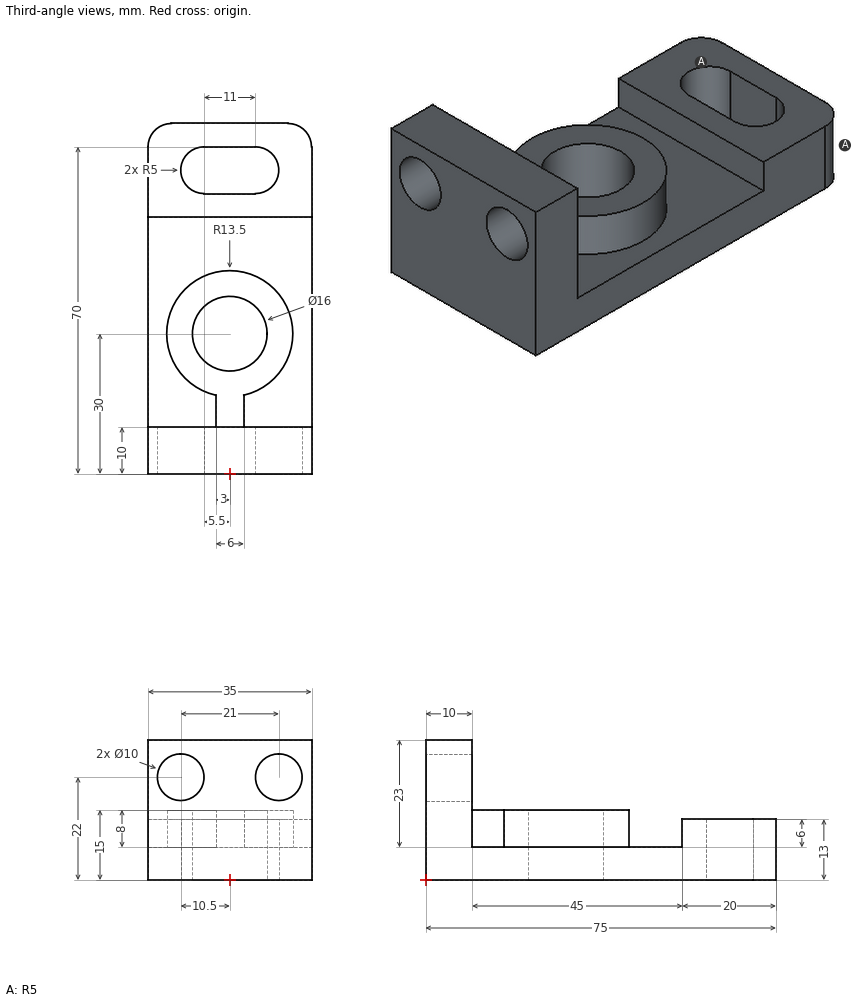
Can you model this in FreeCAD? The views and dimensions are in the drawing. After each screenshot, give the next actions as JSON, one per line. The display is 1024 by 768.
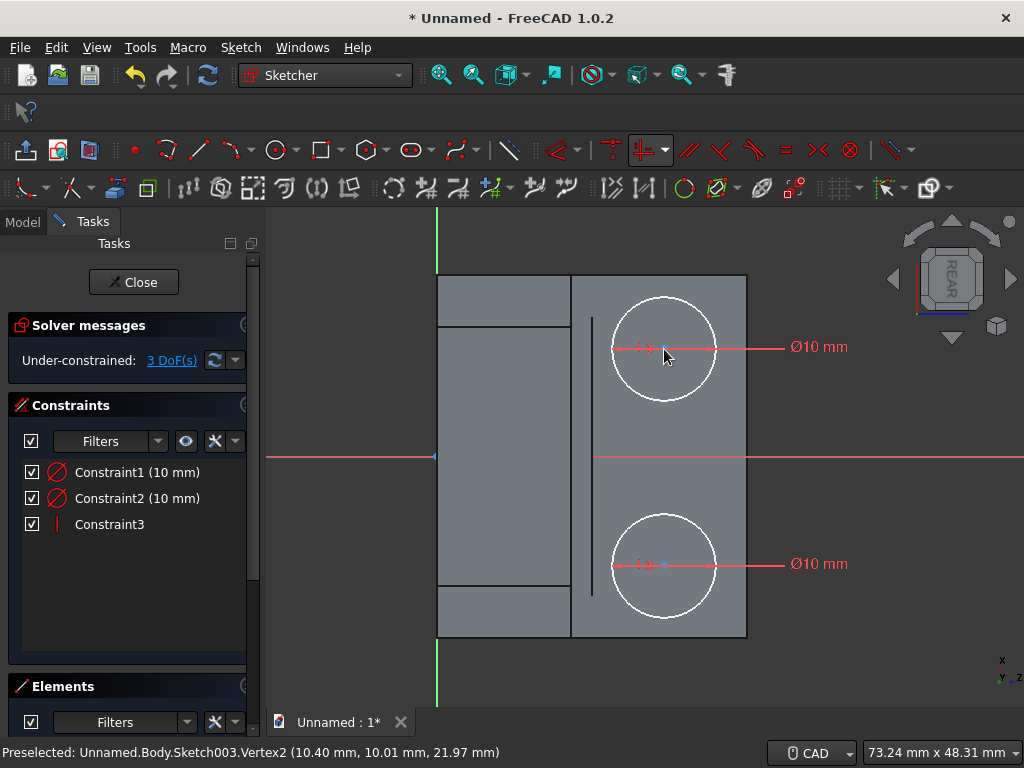
{"action": "key", "text": "d"}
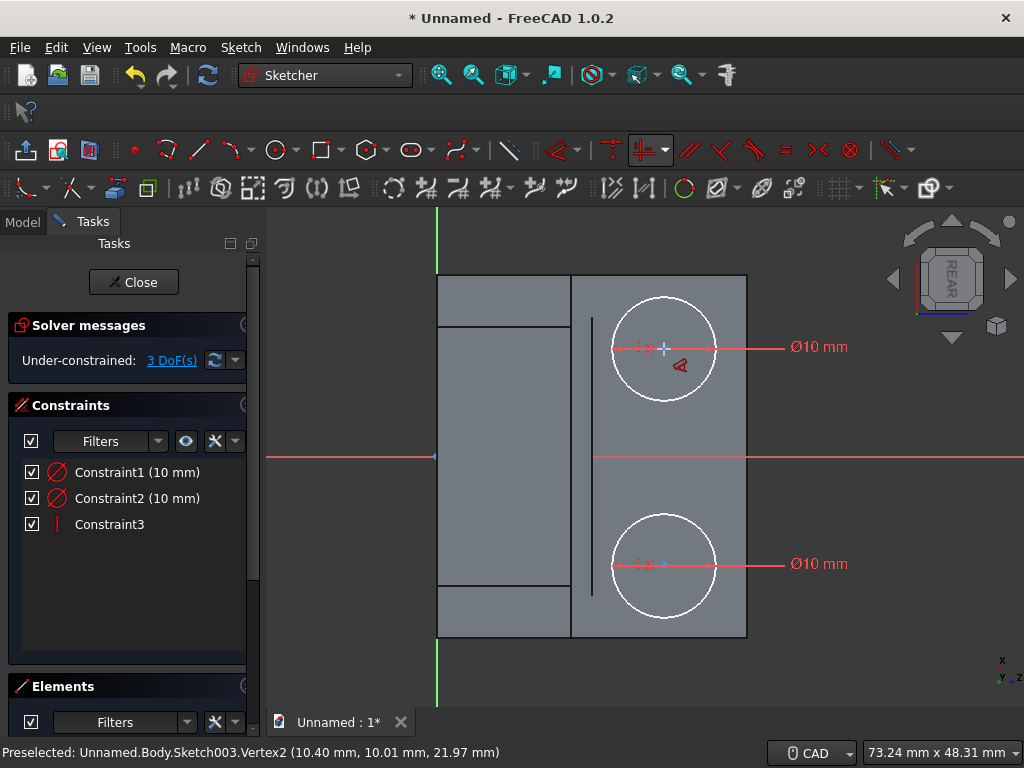
{"action": "left_click", "coordinate": [664, 566]}
{"action": "left_click", "coordinate": [550, 600]}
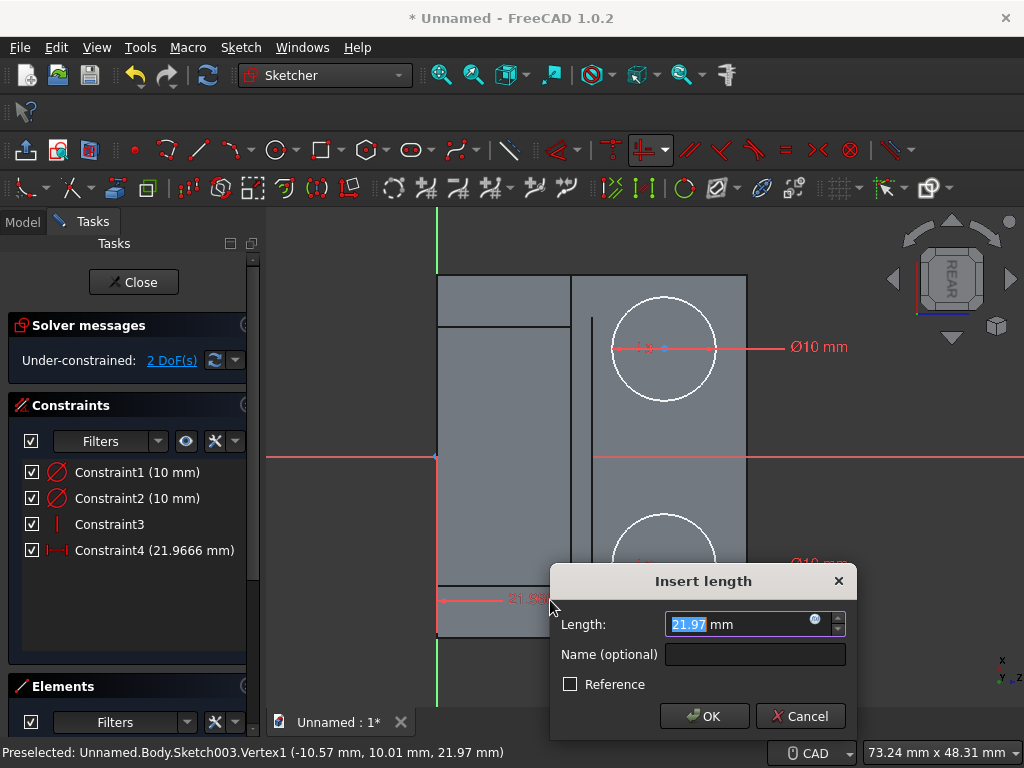
{"action": "type", "text": "22"}
{"action": "key", "text": "Return"}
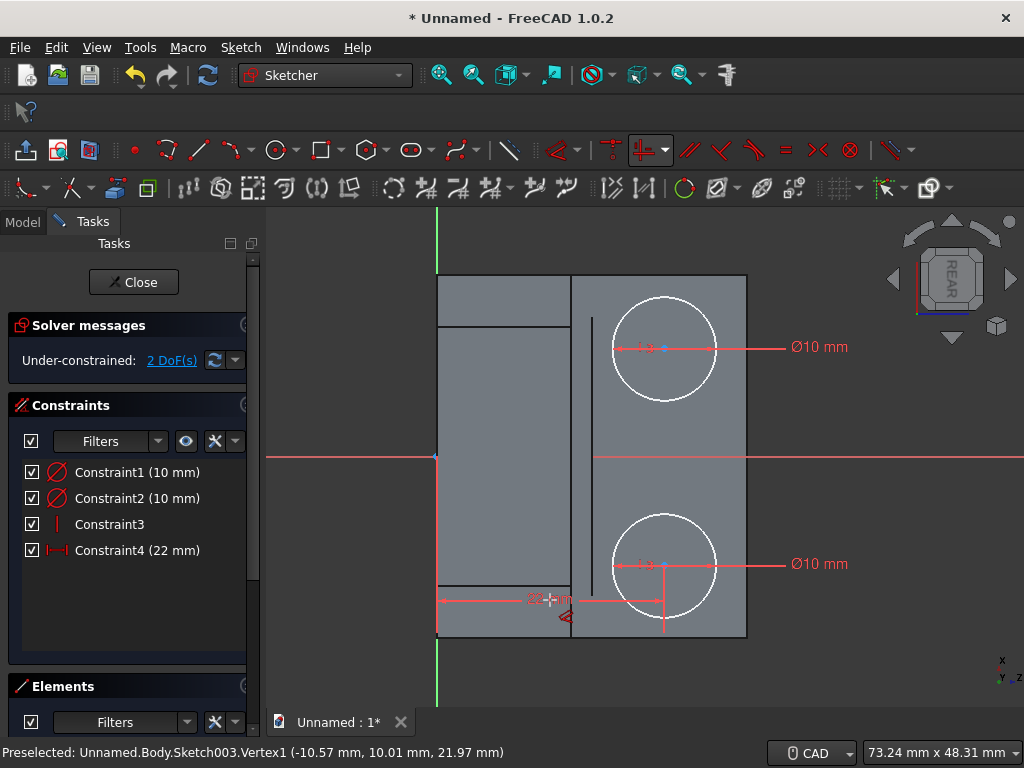
{"action": "left_click", "coordinate": [664, 566]}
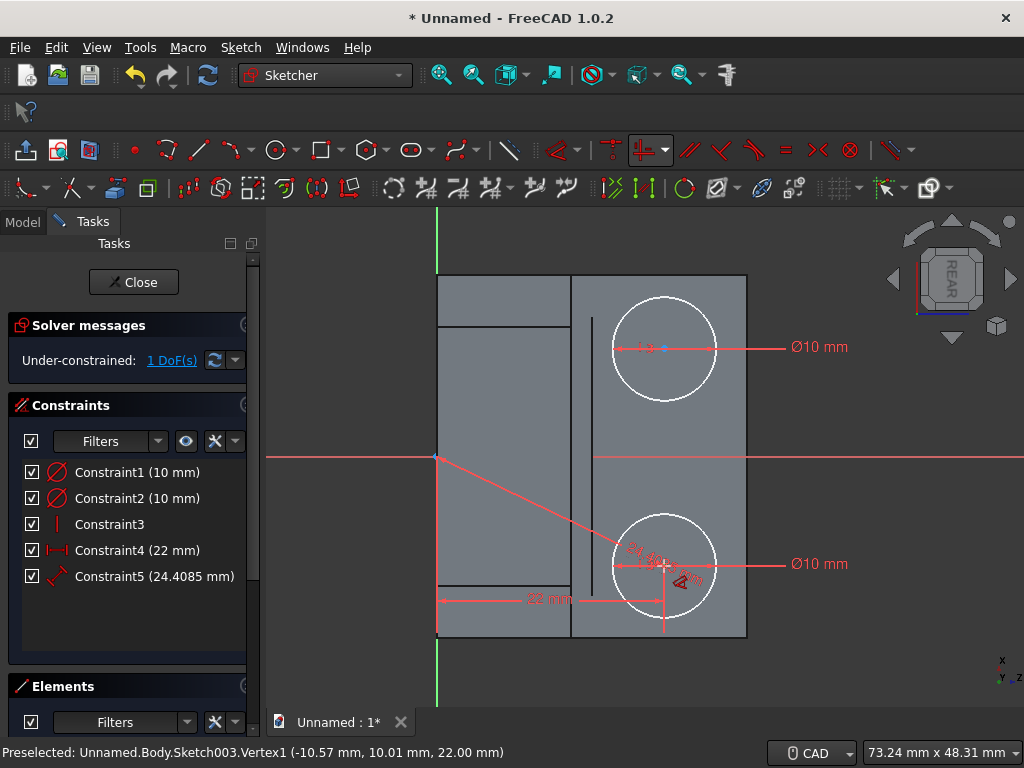
{"action": "left_click", "coordinate": [664, 349]}
{"action": "left_click", "coordinate": [698, 408]}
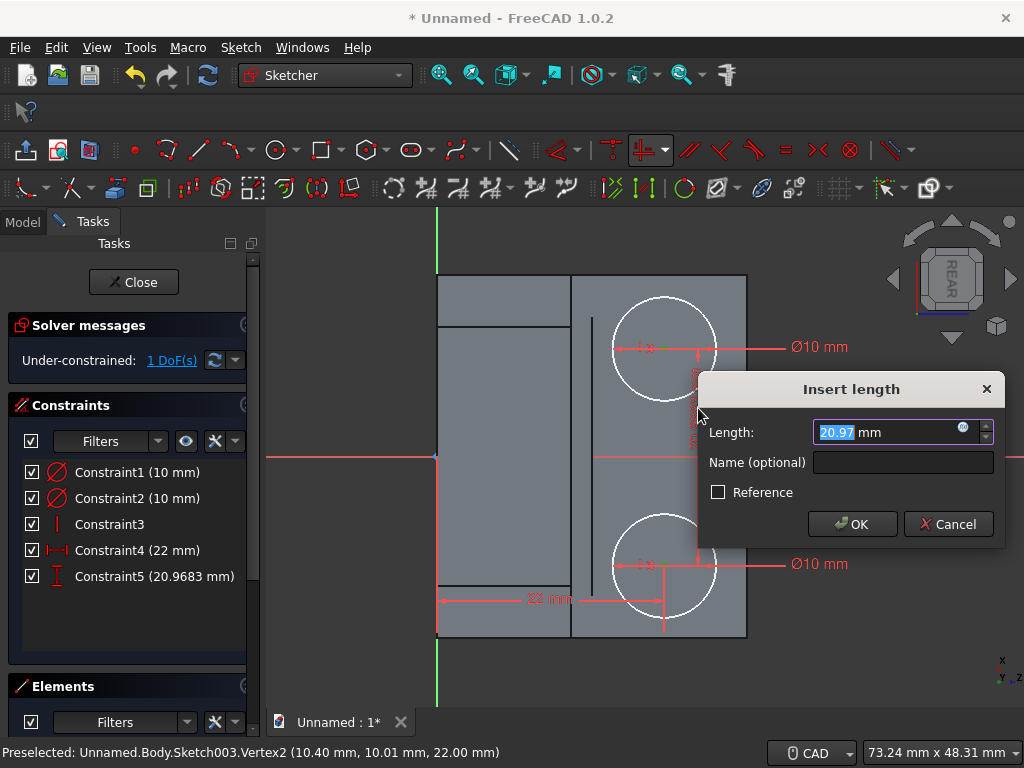
{"action": "type", "text": "21"}
{"action": "key", "text": "Return"}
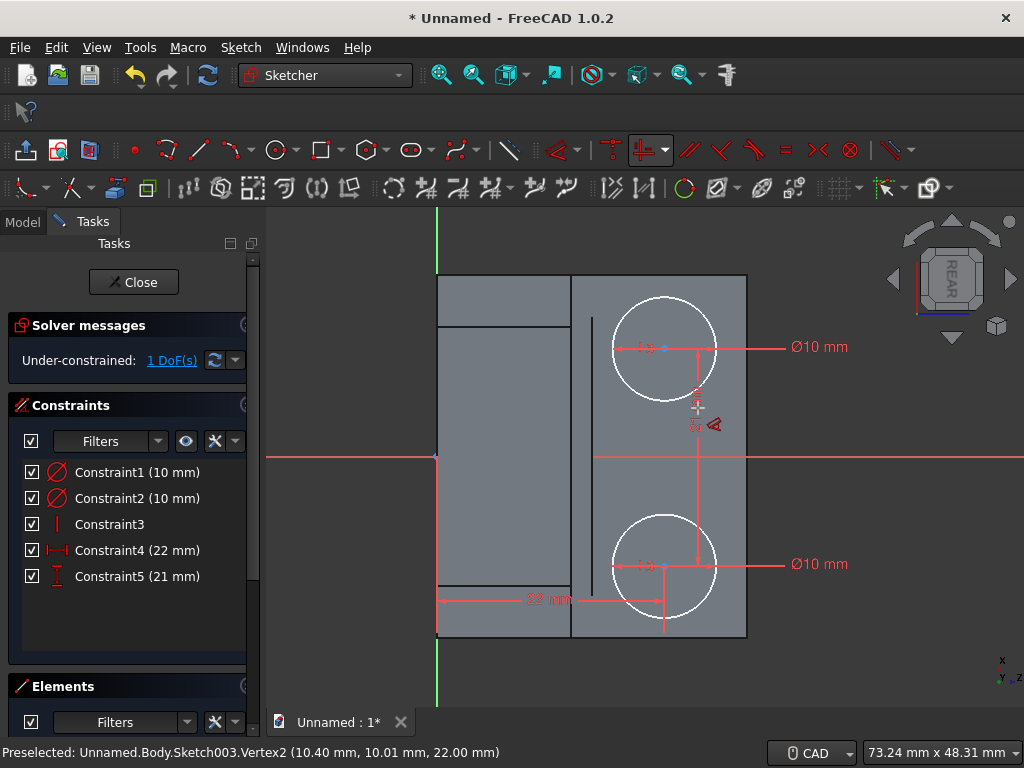
{"action": "left_click", "coordinate": [664, 566]}
{"action": "left_click", "coordinate": [403, 511]}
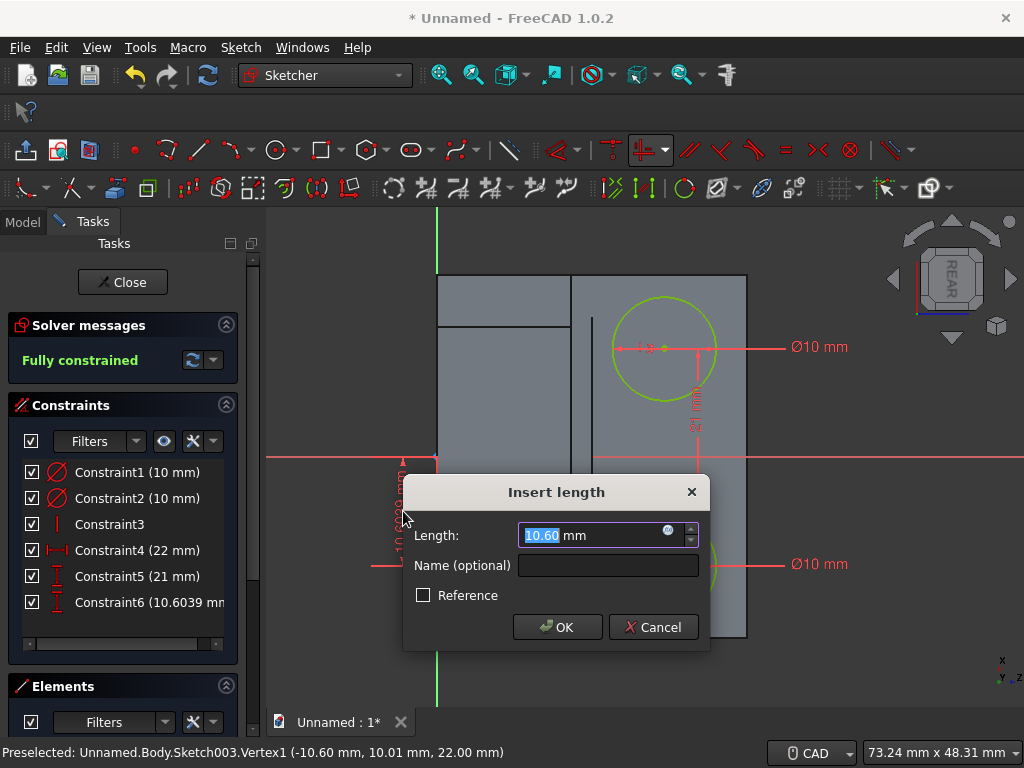
{"action": "type", "text": "10.5"}
{"action": "key", "text": "Return"}
{"action": "key", "text": "Escape"}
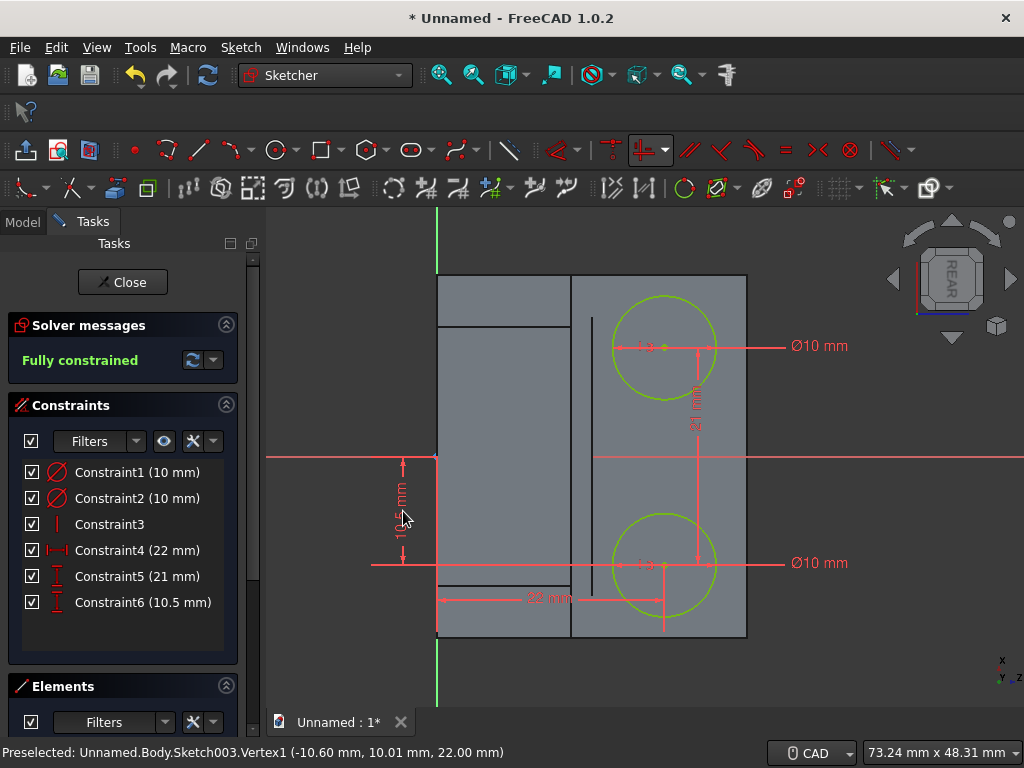
{"action": "left_click", "coordinate": [123, 282]}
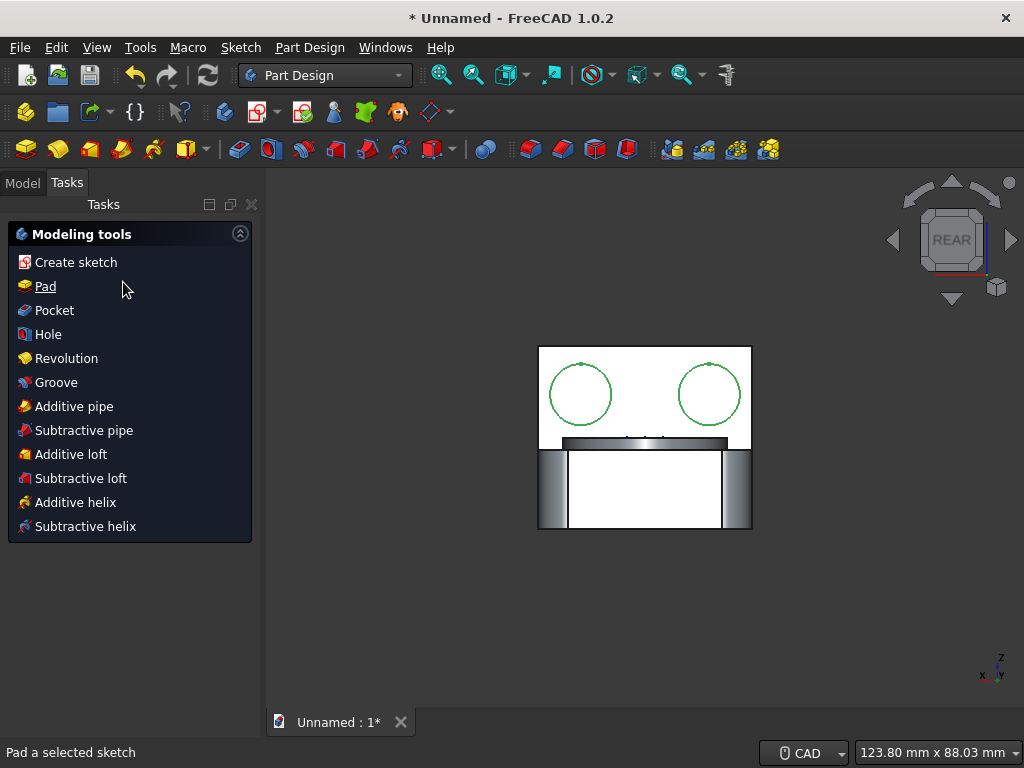
{"action": "left_click", "coordinate": [240, 150]}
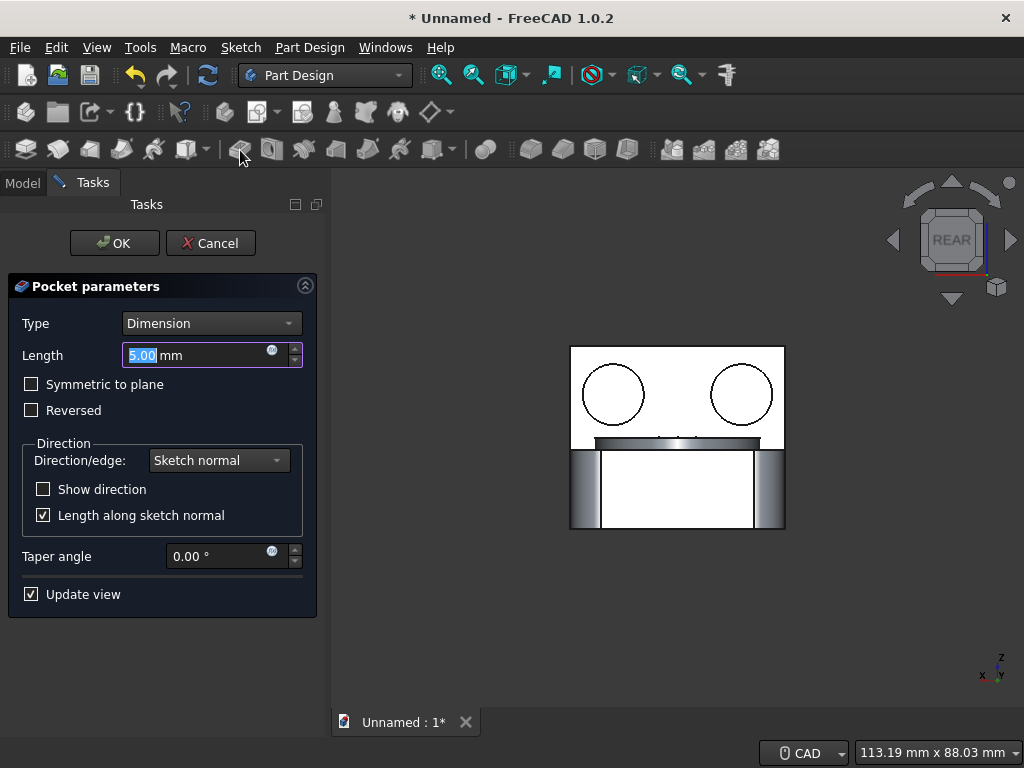
{"action": "type", "text": "10"}
{"action": "key", "text": "Tab"}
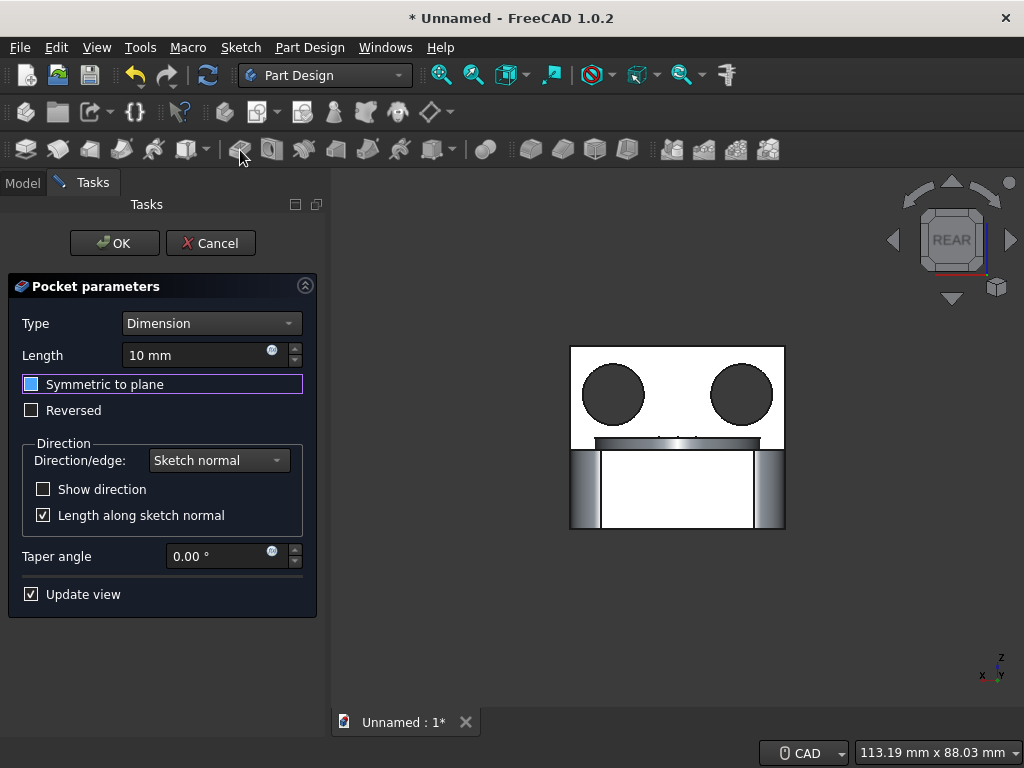
{"action": "left_click", "coordinate": [115, 243]}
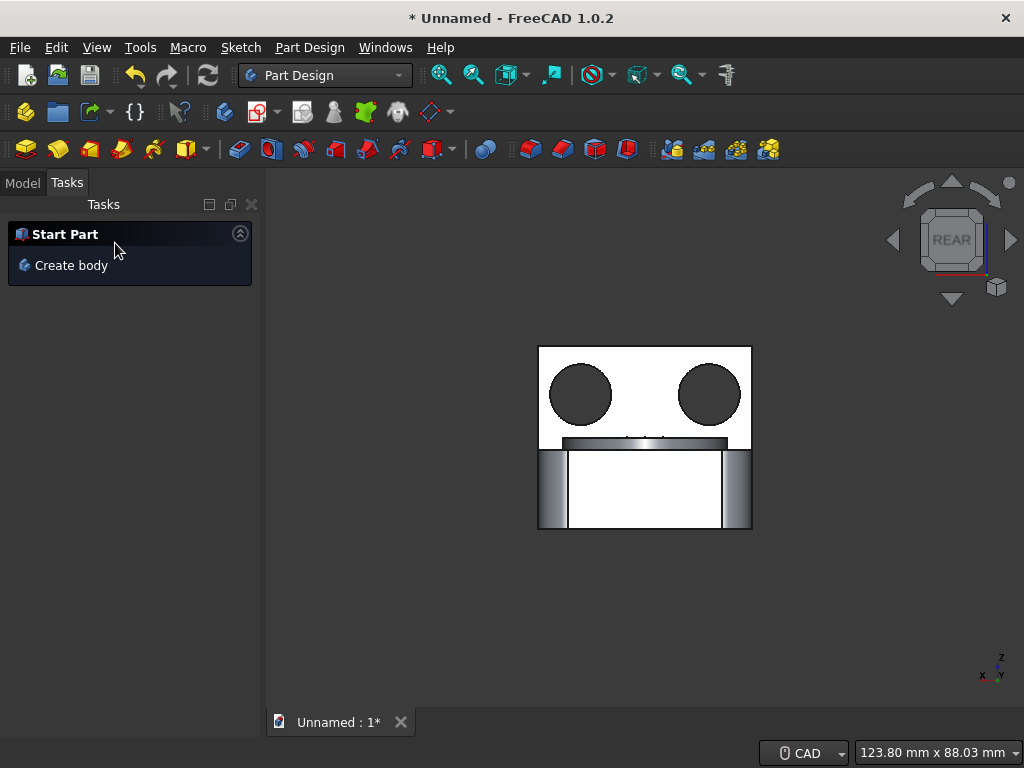
{"action": "key", "text": "0"}